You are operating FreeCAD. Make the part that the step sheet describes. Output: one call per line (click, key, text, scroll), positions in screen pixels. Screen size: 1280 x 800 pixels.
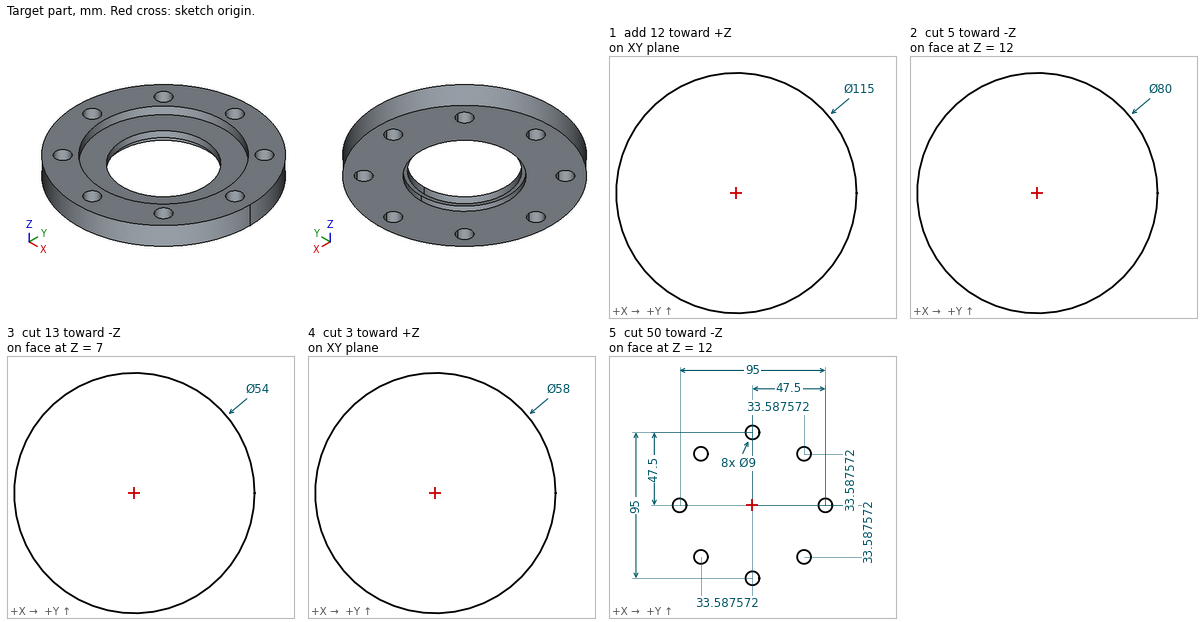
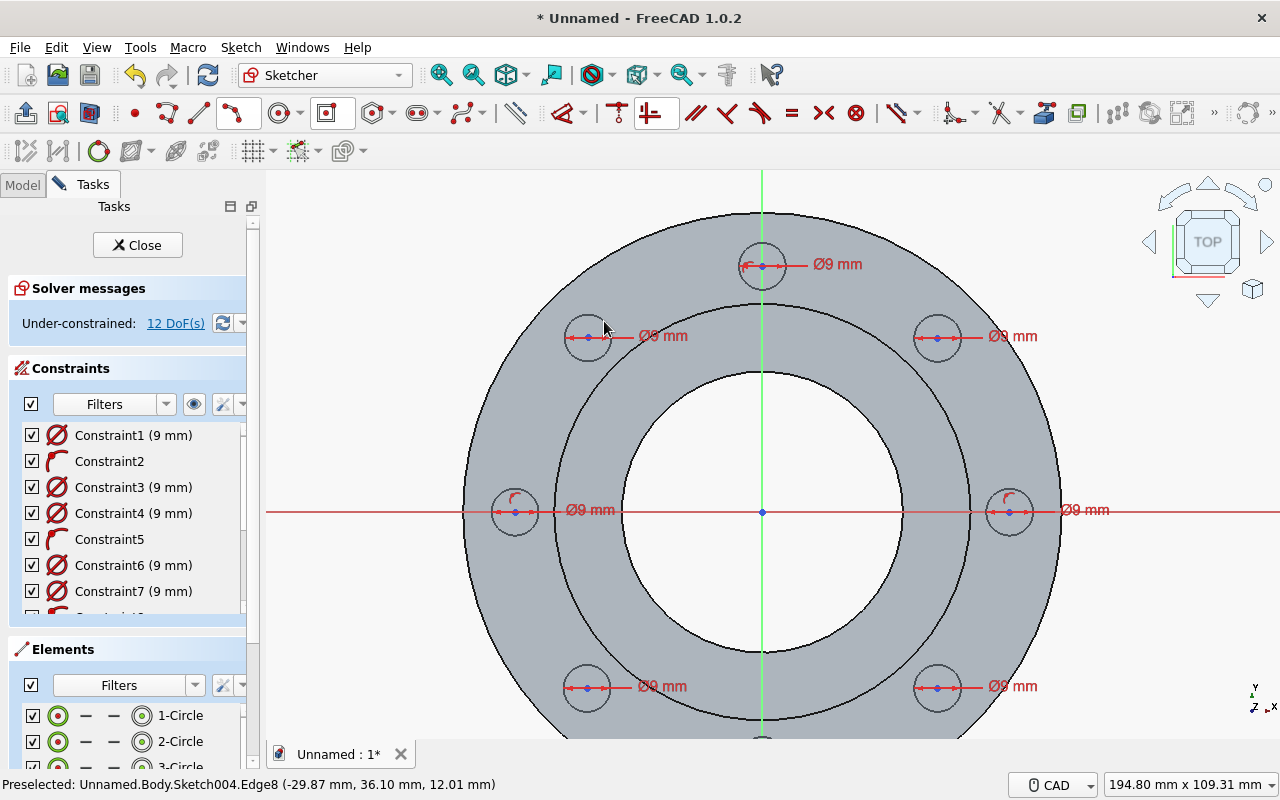
click(938, 338)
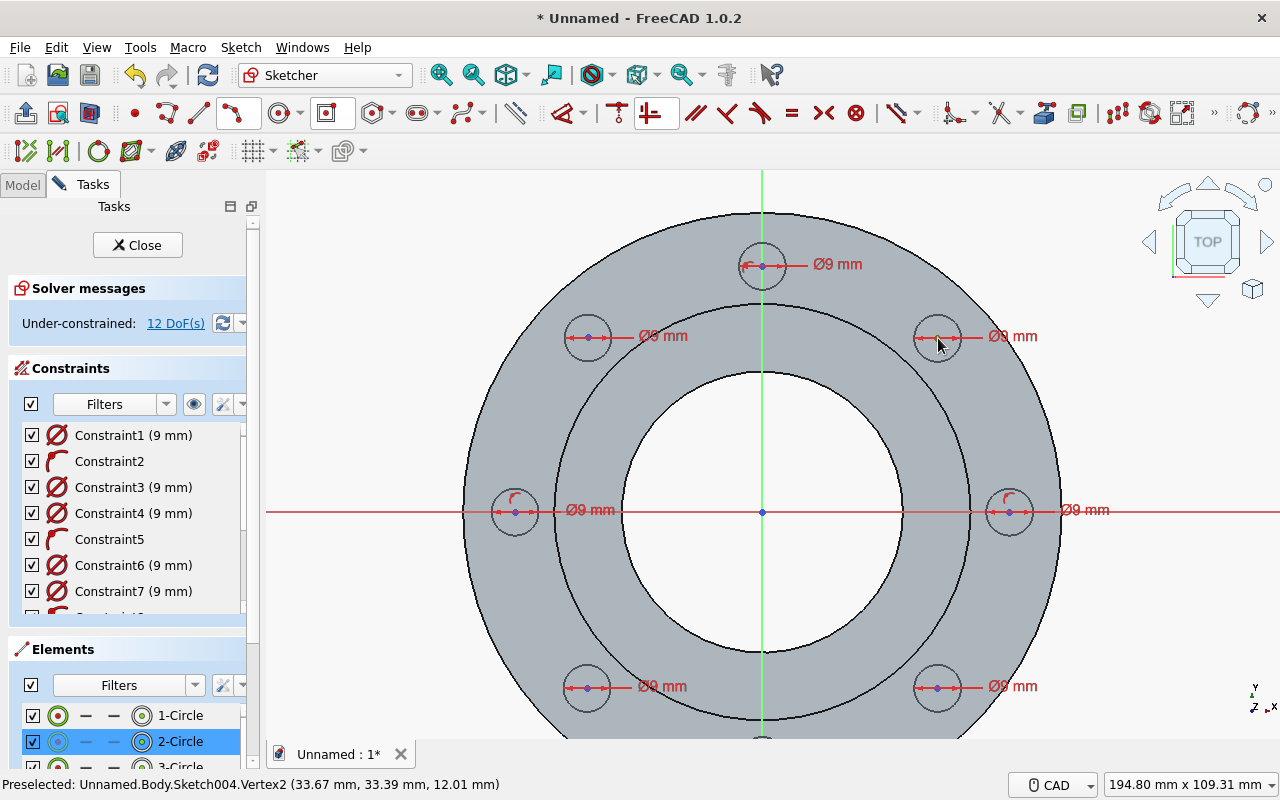
click(938, 688)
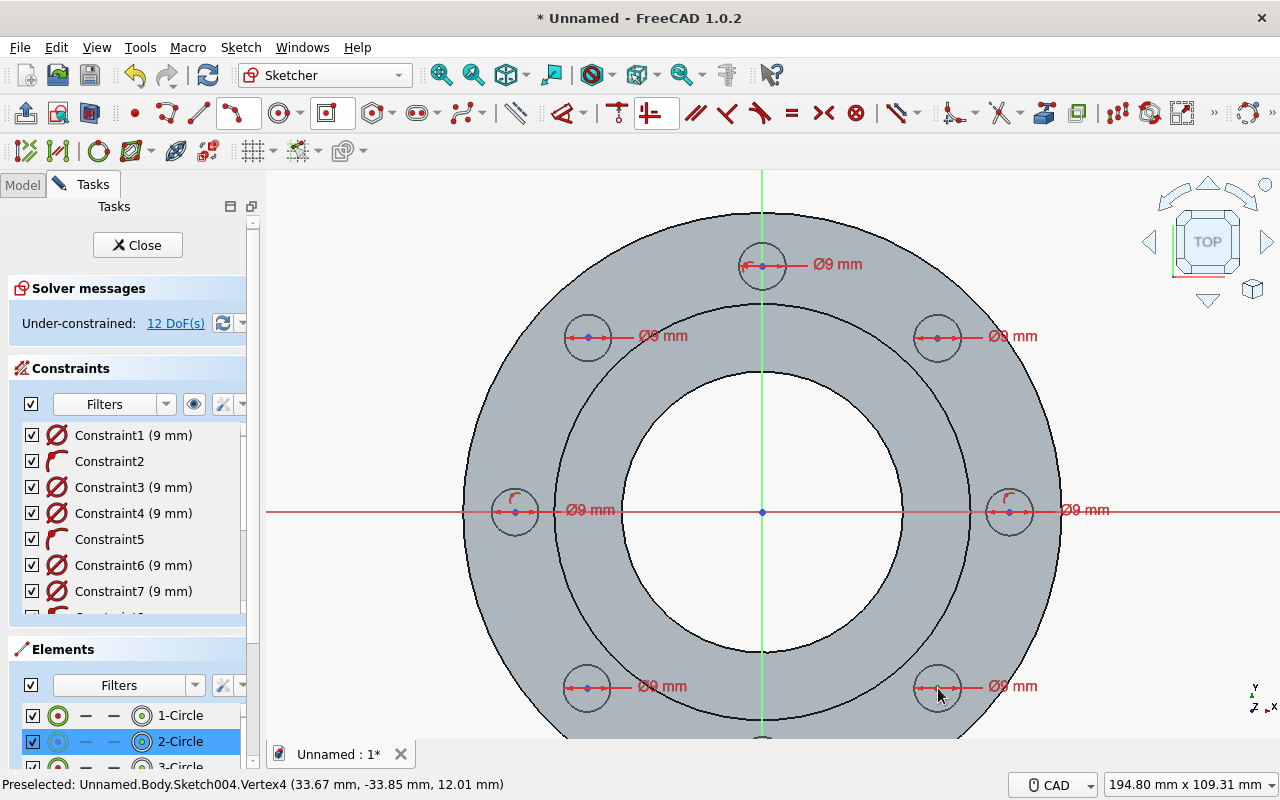
key(v)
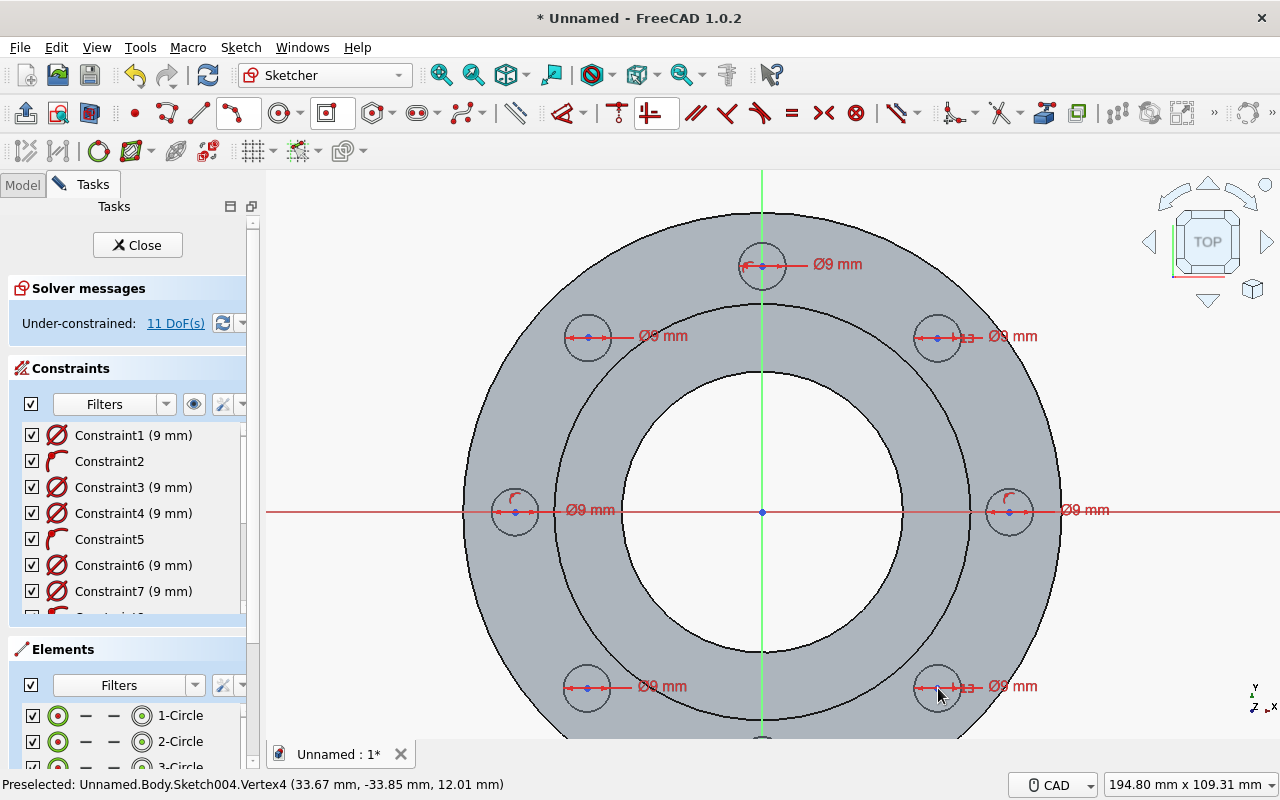
click(938, 688)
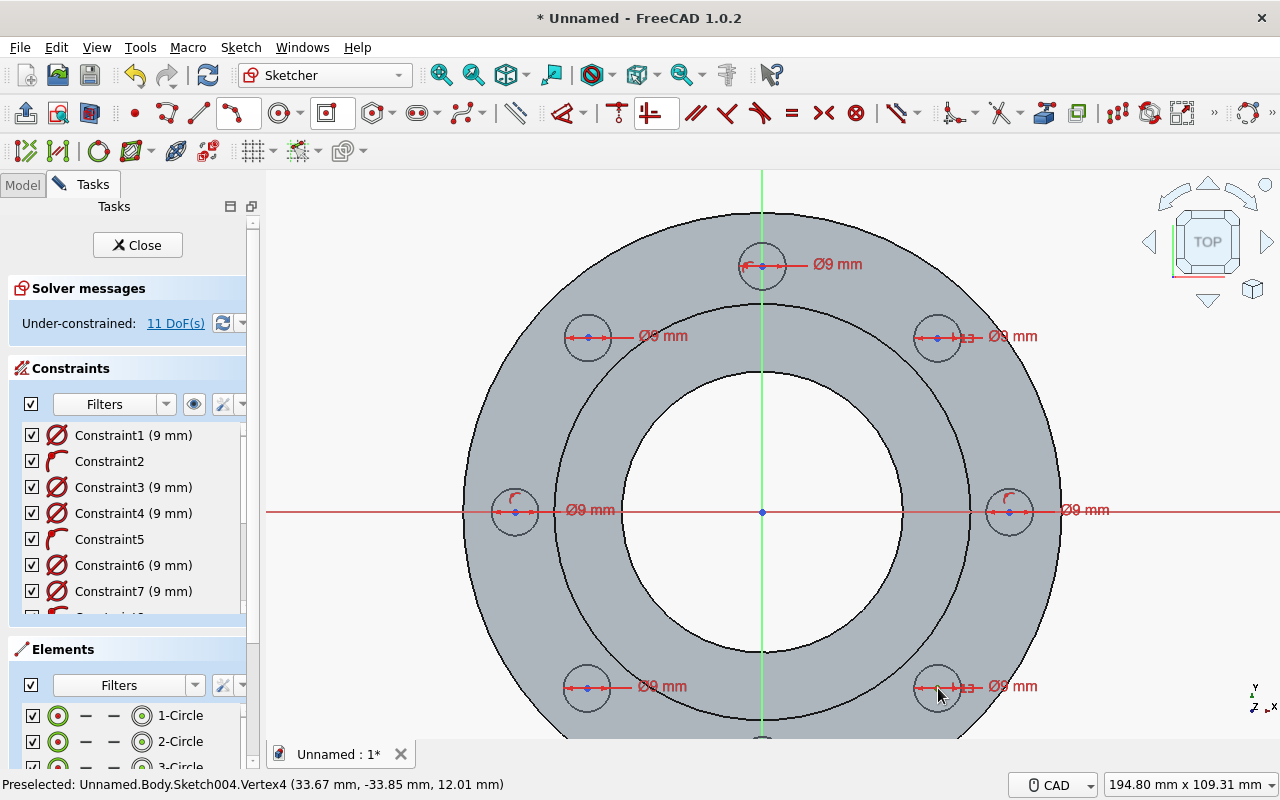
click(587, 688)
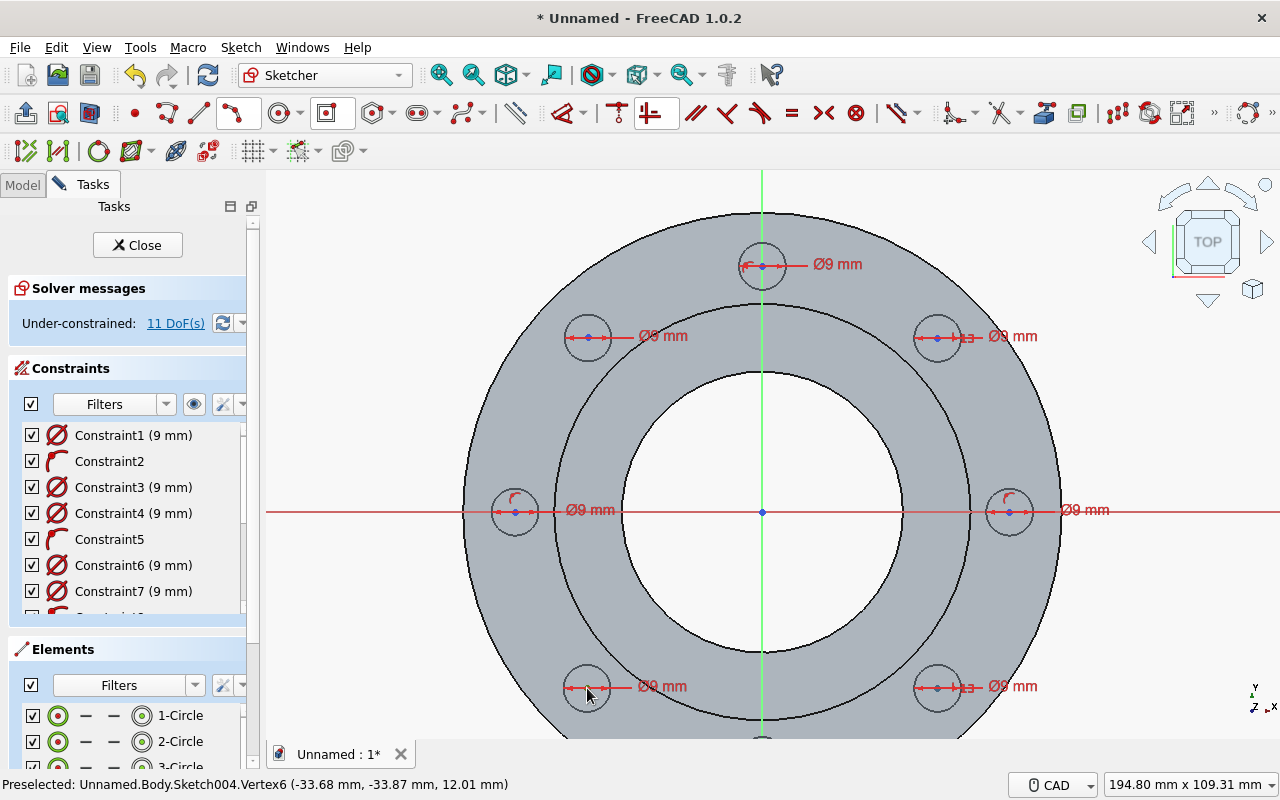
click(674, 114)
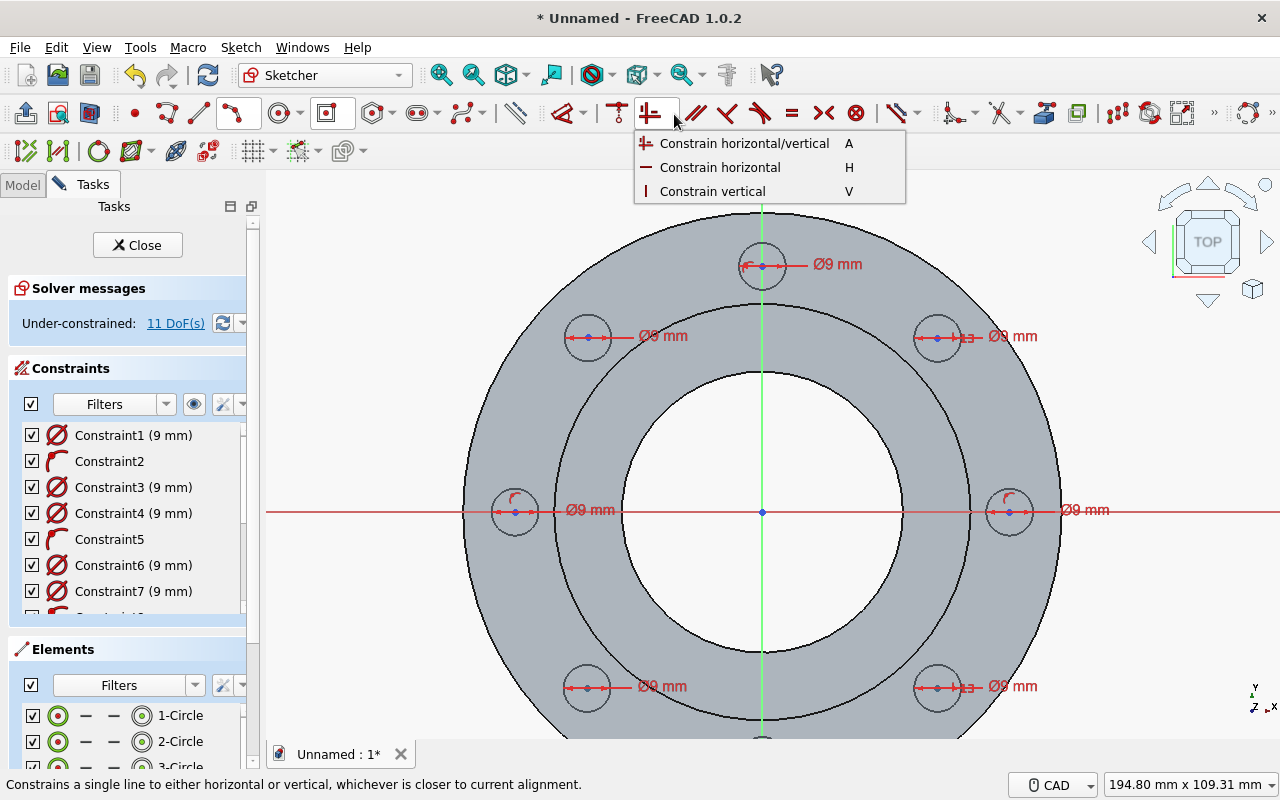
click(770, 167)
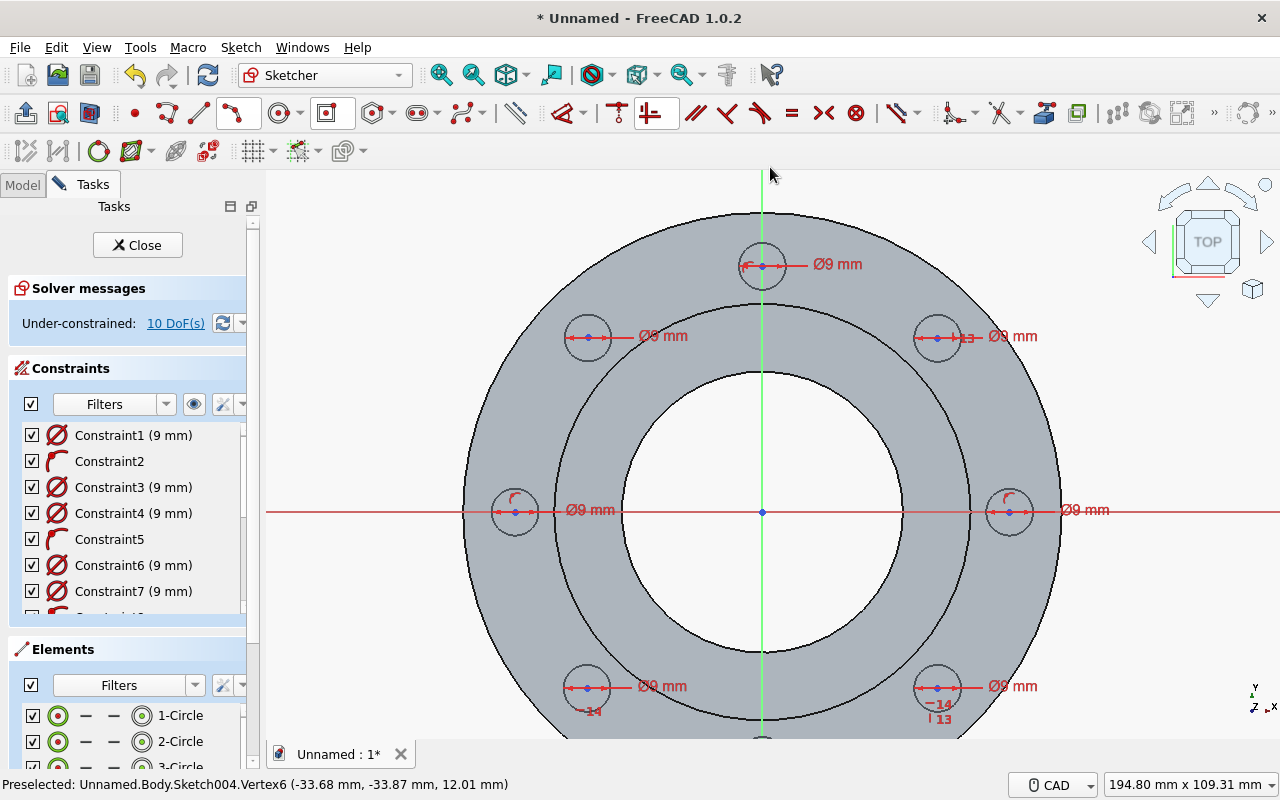
click(587, 688)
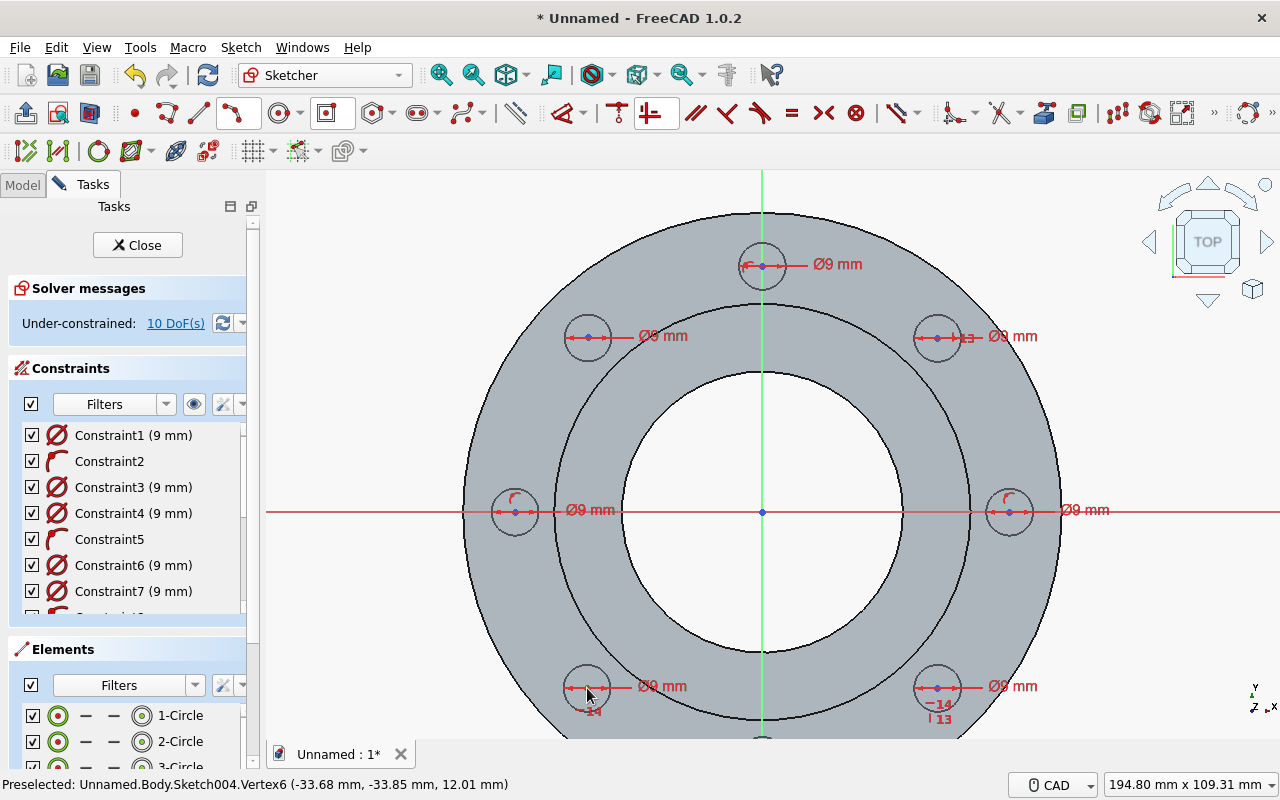
click(588, 338)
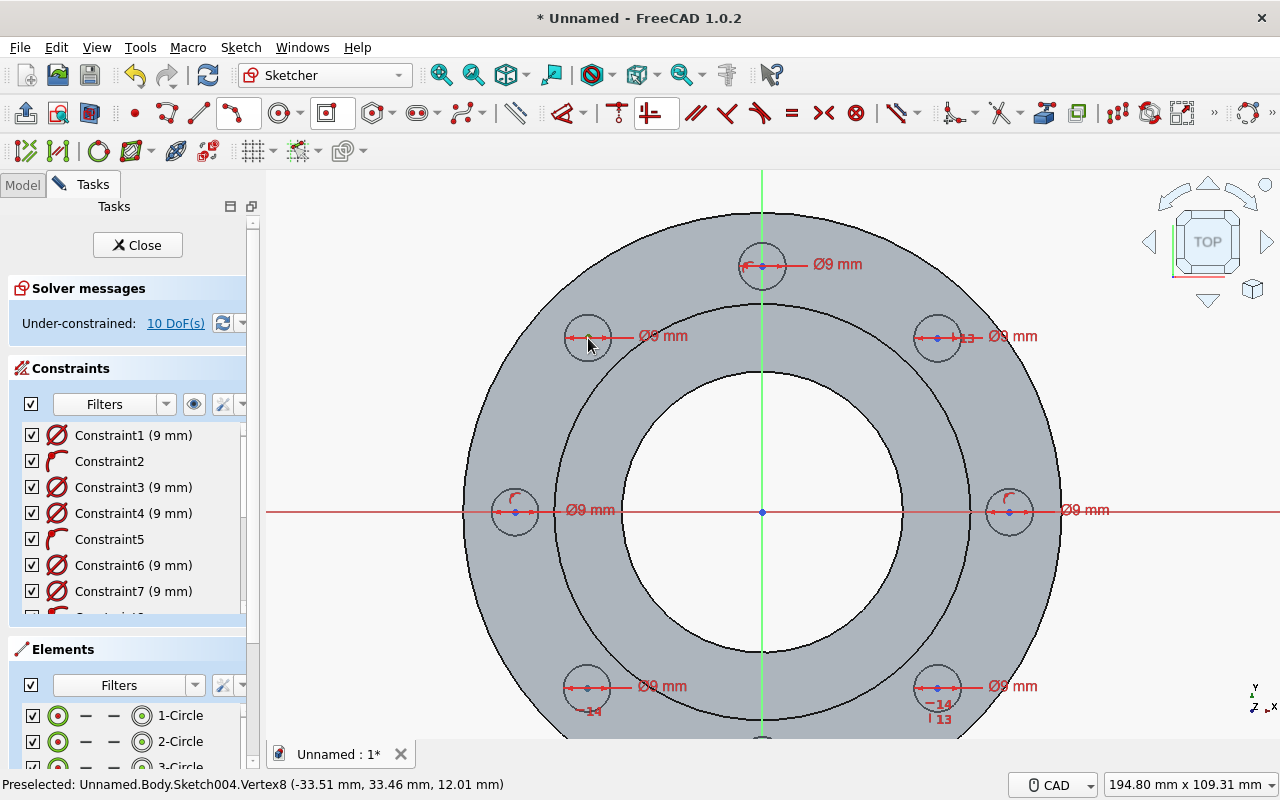
click(674, 114)